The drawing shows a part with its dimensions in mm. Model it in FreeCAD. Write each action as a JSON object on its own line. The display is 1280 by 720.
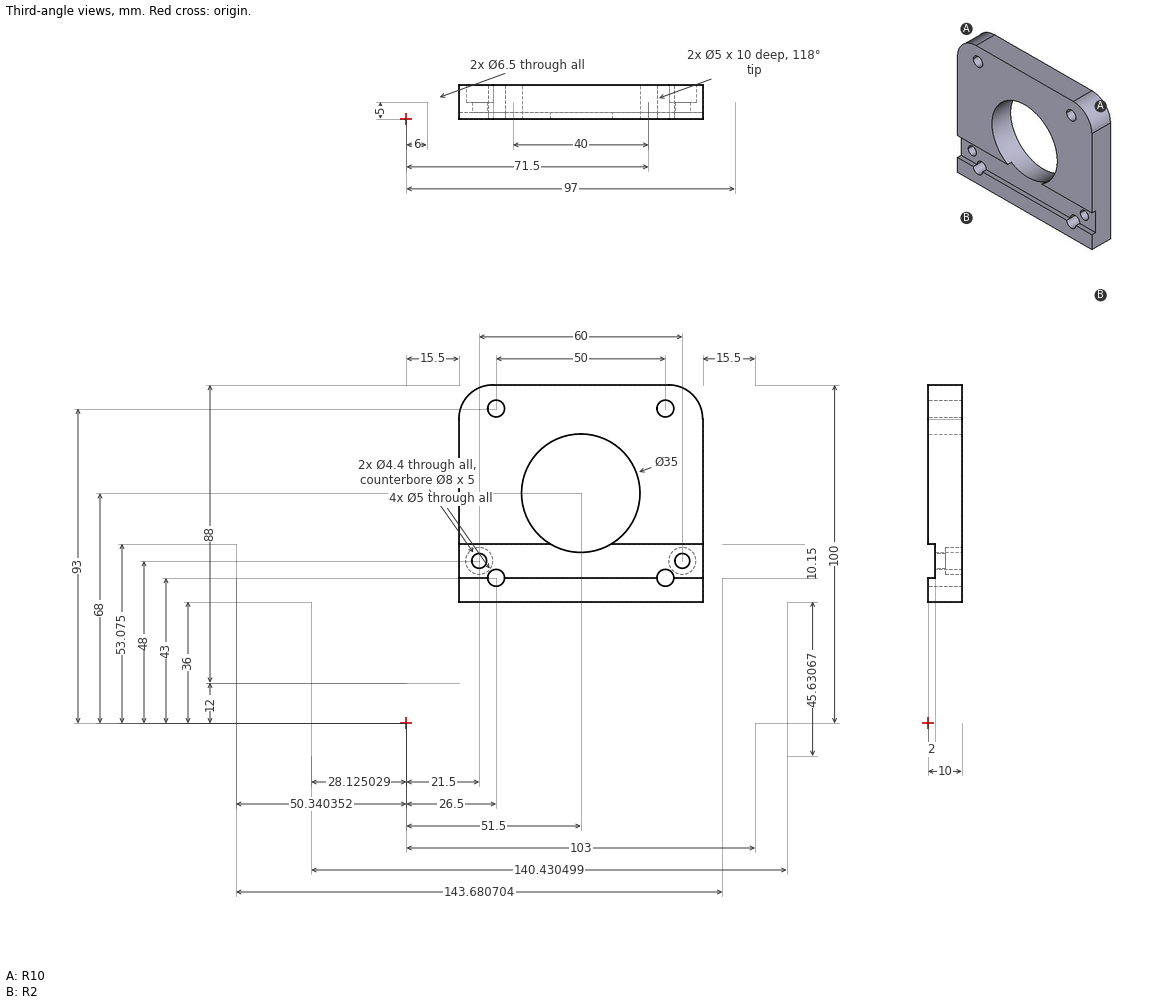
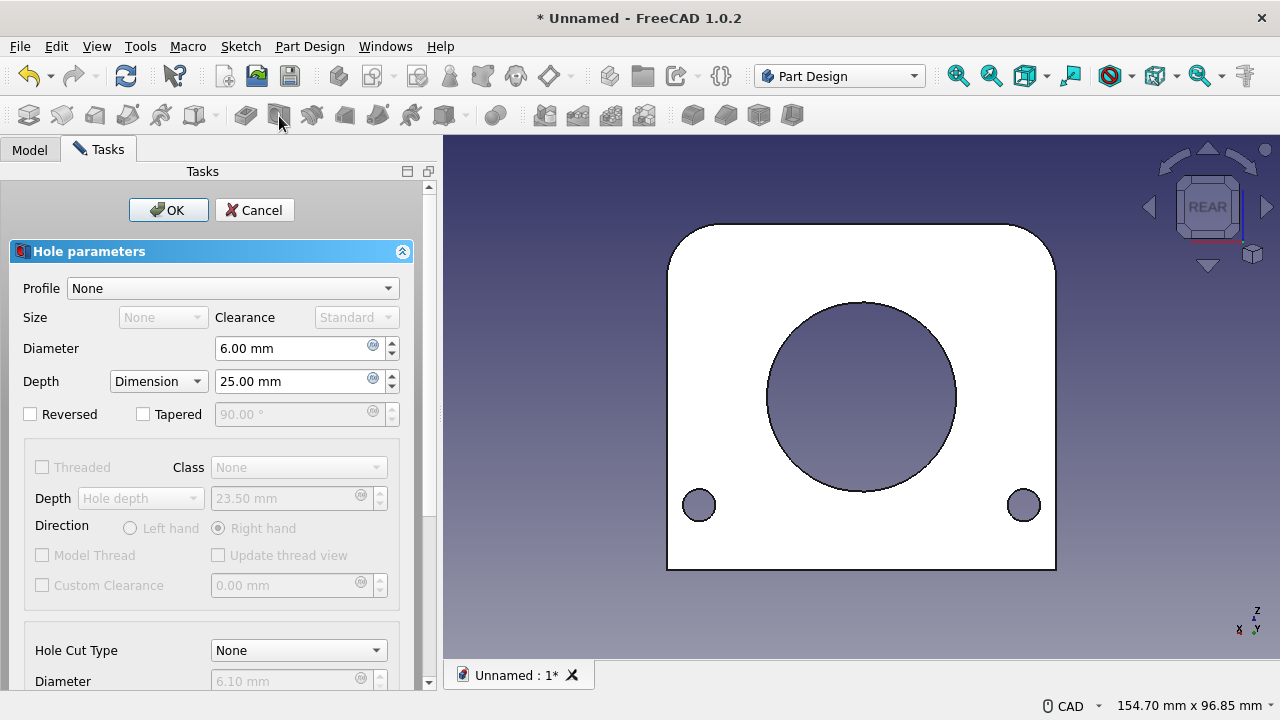
{"action": "triple_click", "coordinate": [300, 348]}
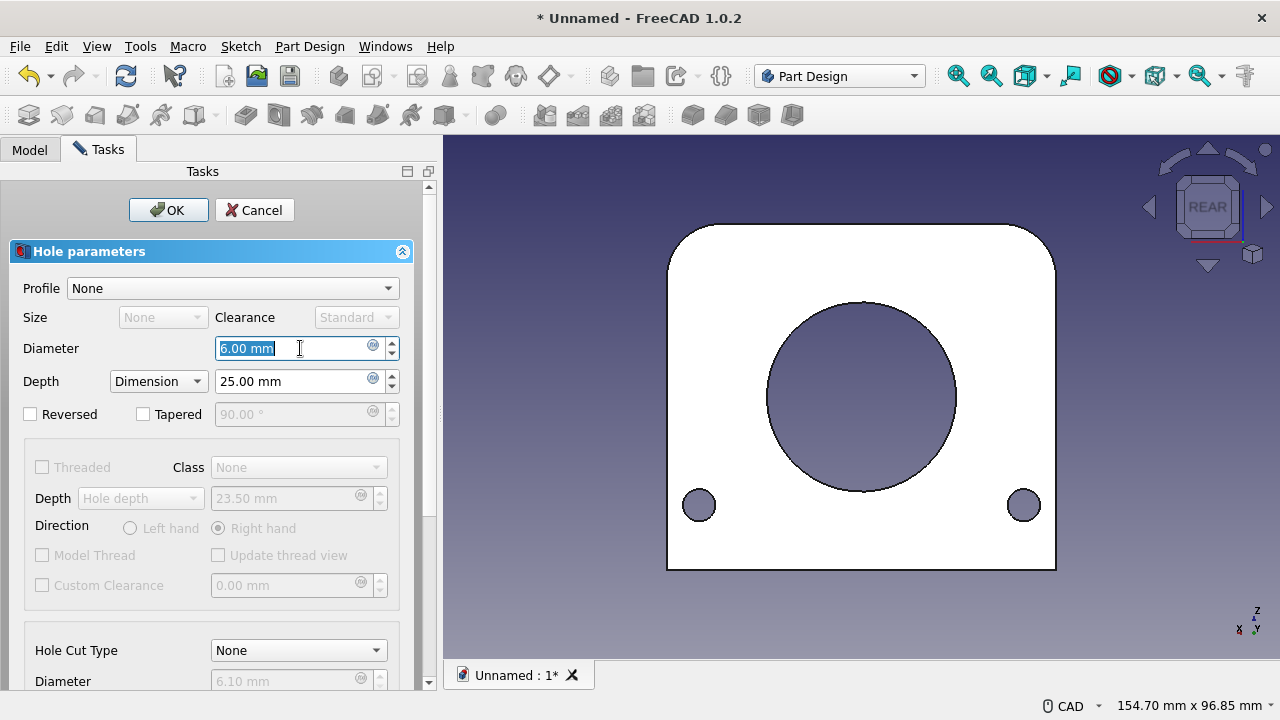
{"action": "type", "text": "4.4"}
{"action": "key", "text": "Tab"}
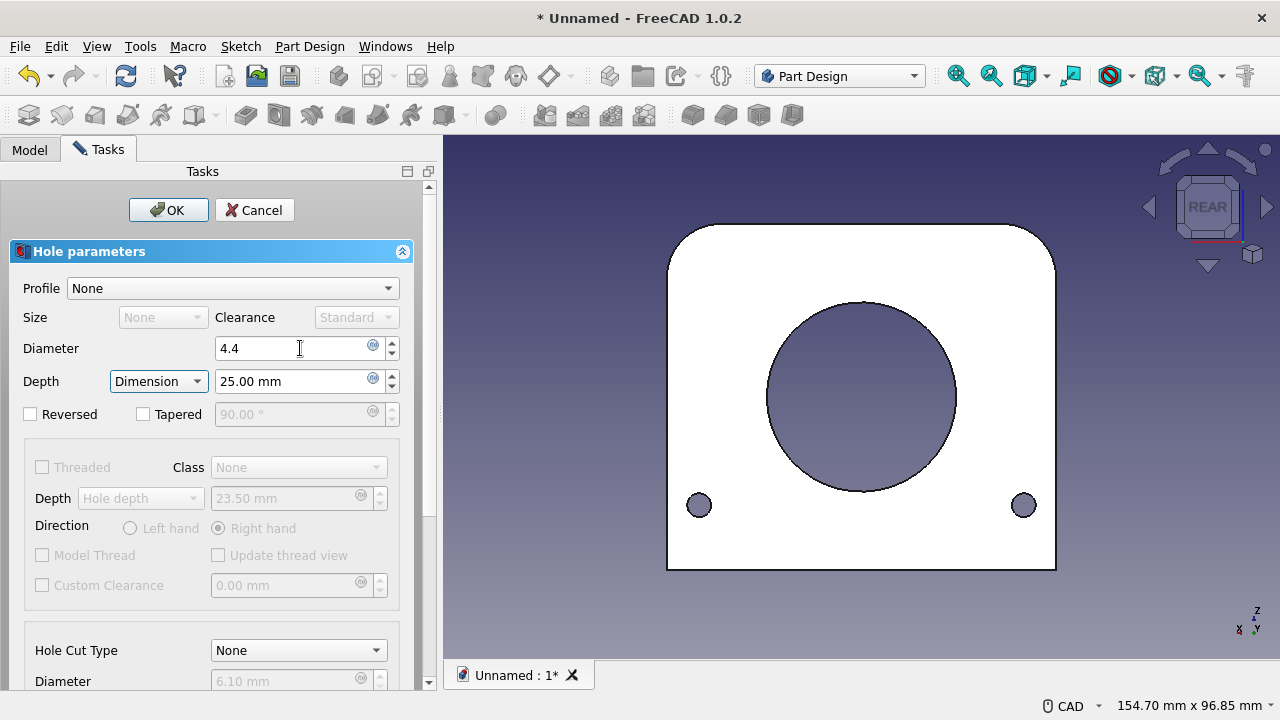
{"action": "left_click", "coordinate": [160, 382]}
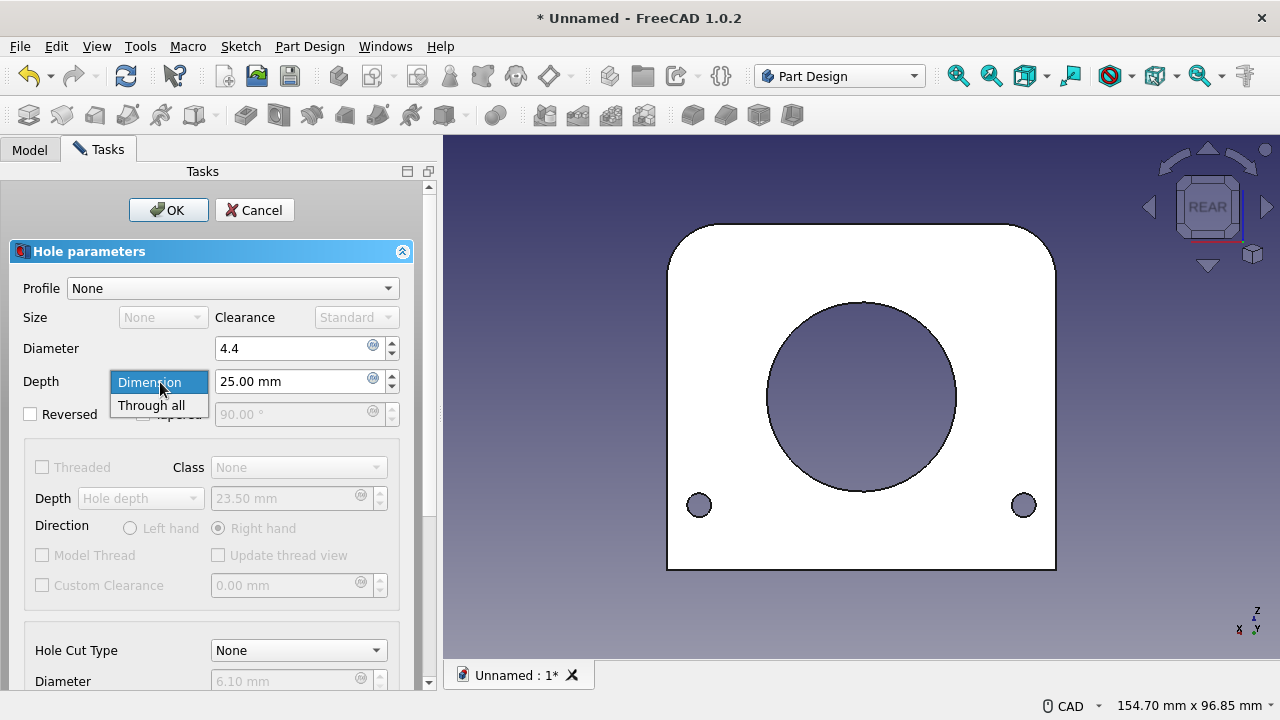
{"action": "left_click", "coordinate": [158, 406]}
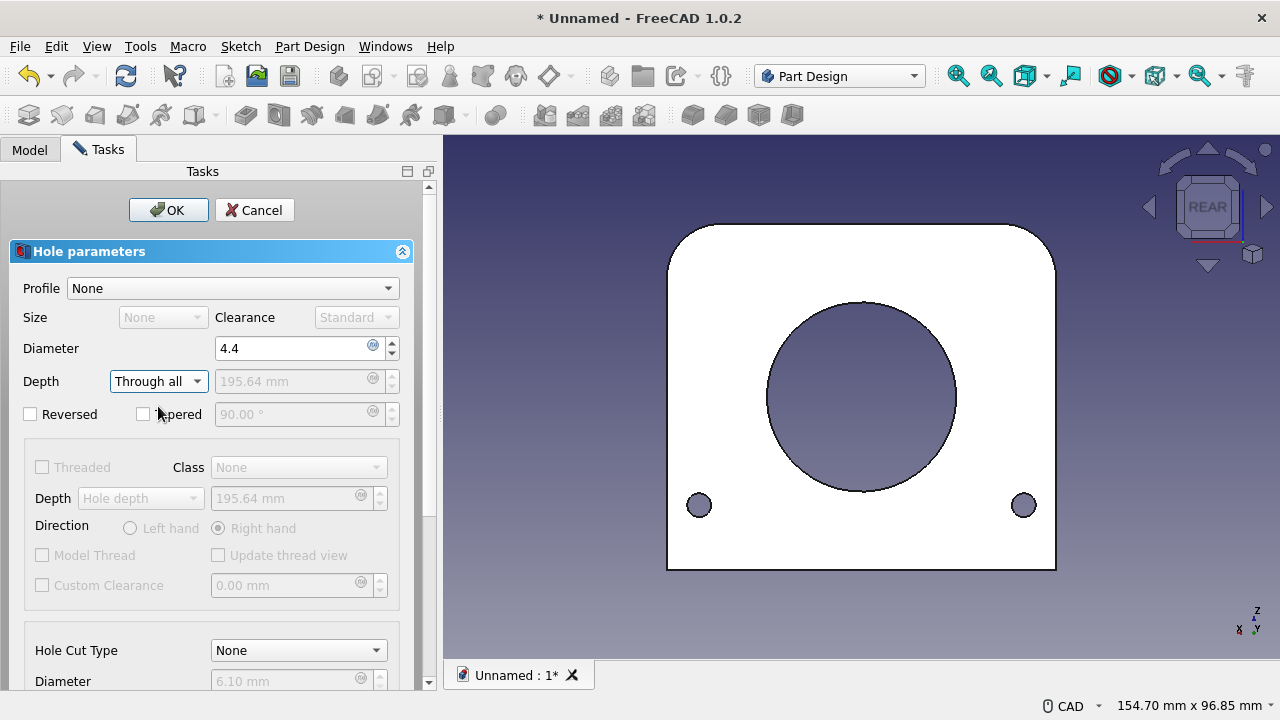
{"action": "left_click", "coordinate": [300, 650]}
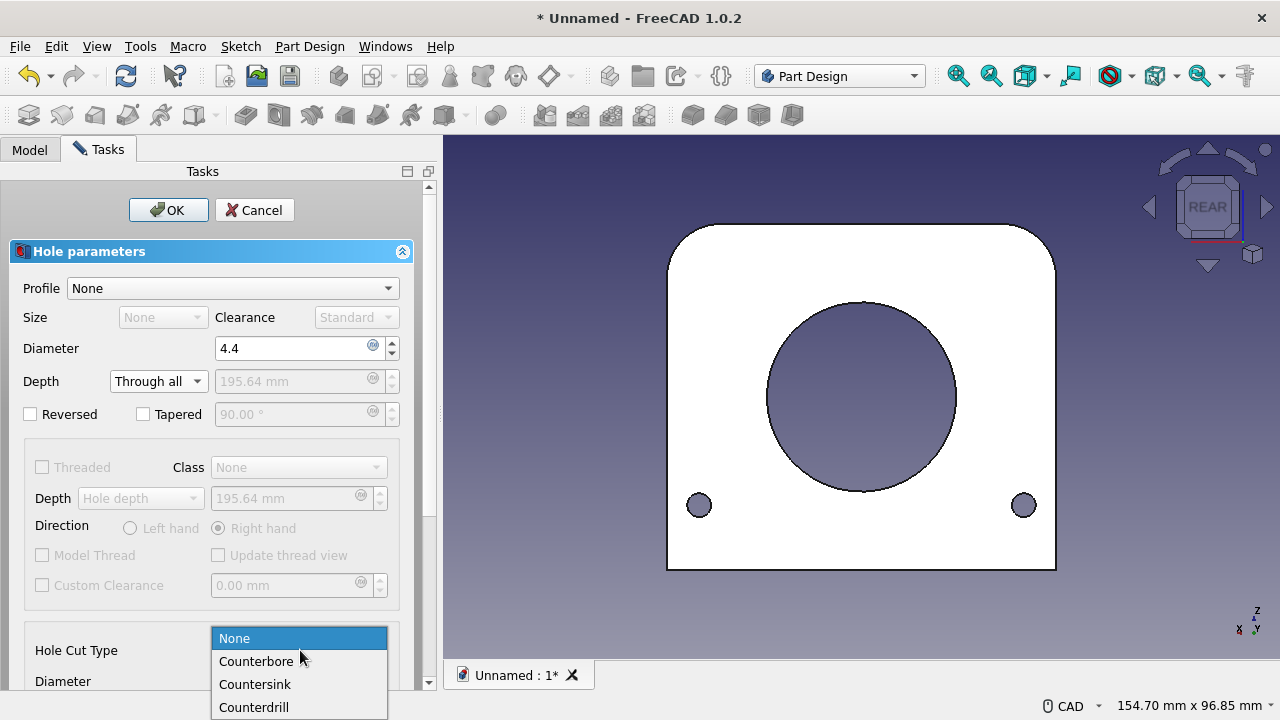
{"action": "left_click", "coordinate": [298, 662]}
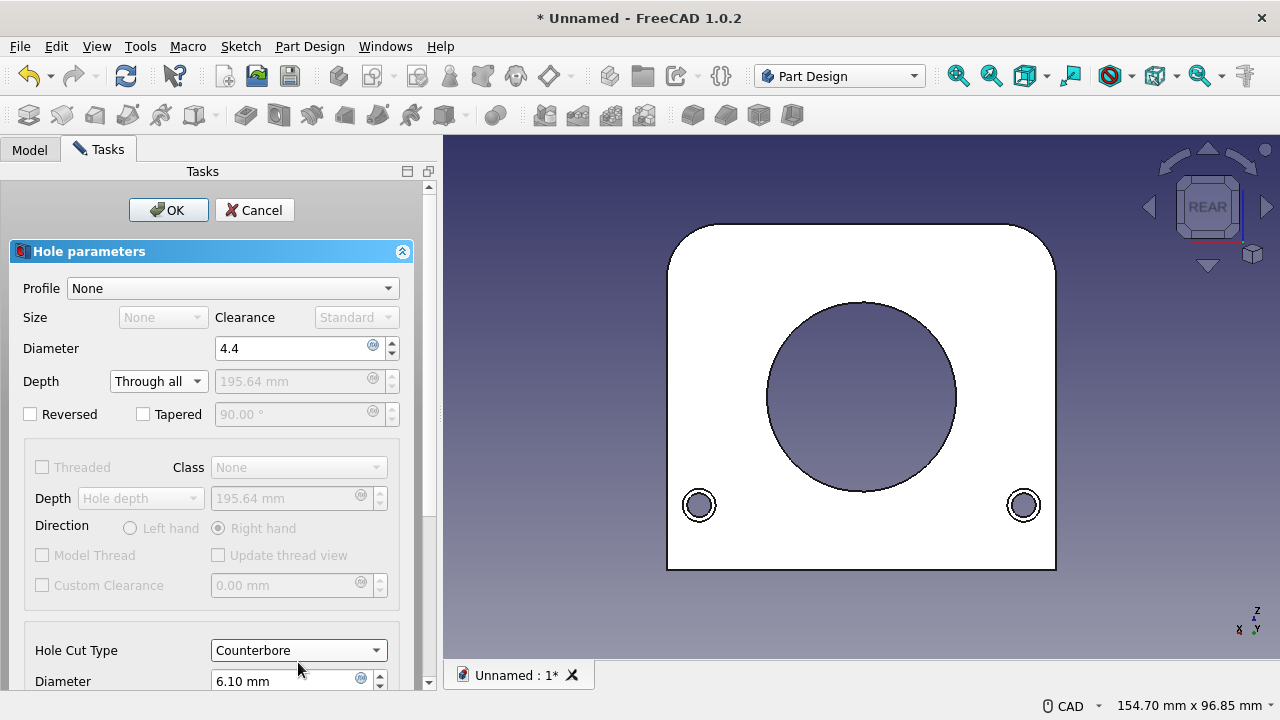
{"action": "scroll", "coordinate": [429, 436], "scroll_direction": "down", "scroll_amount": 2}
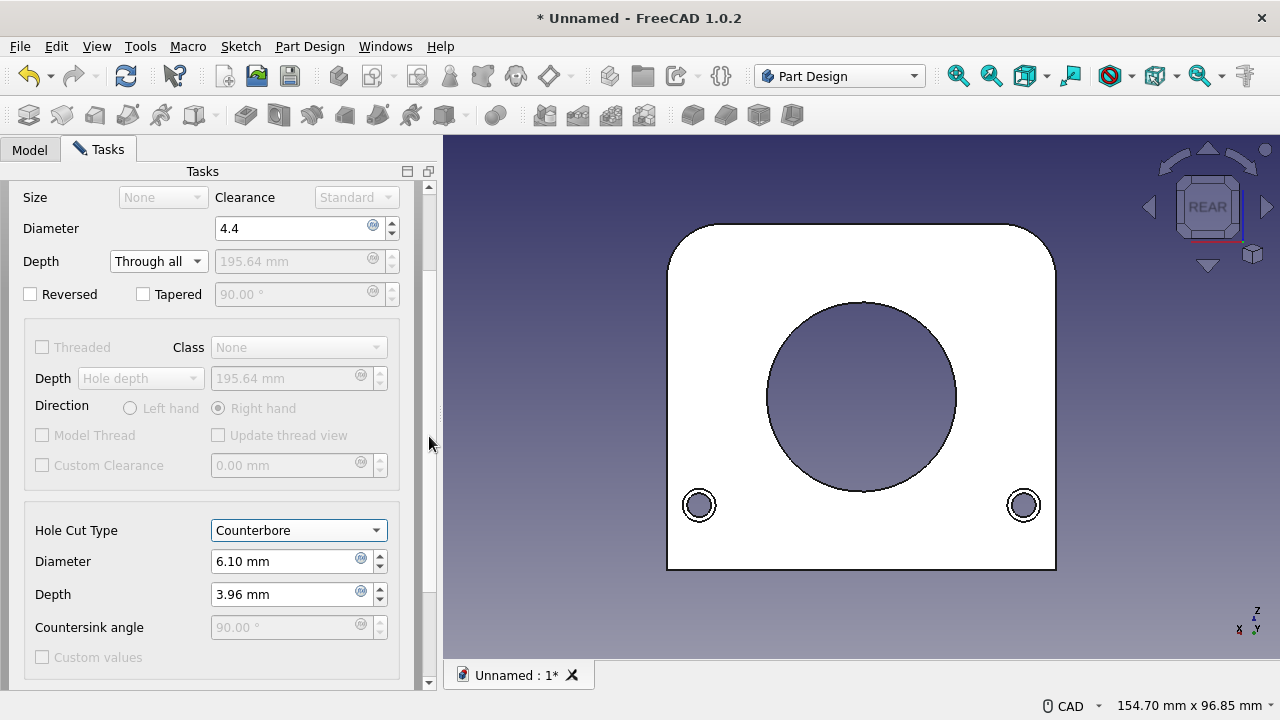
{"action": "triple_click", "coordinate": [292, 562]}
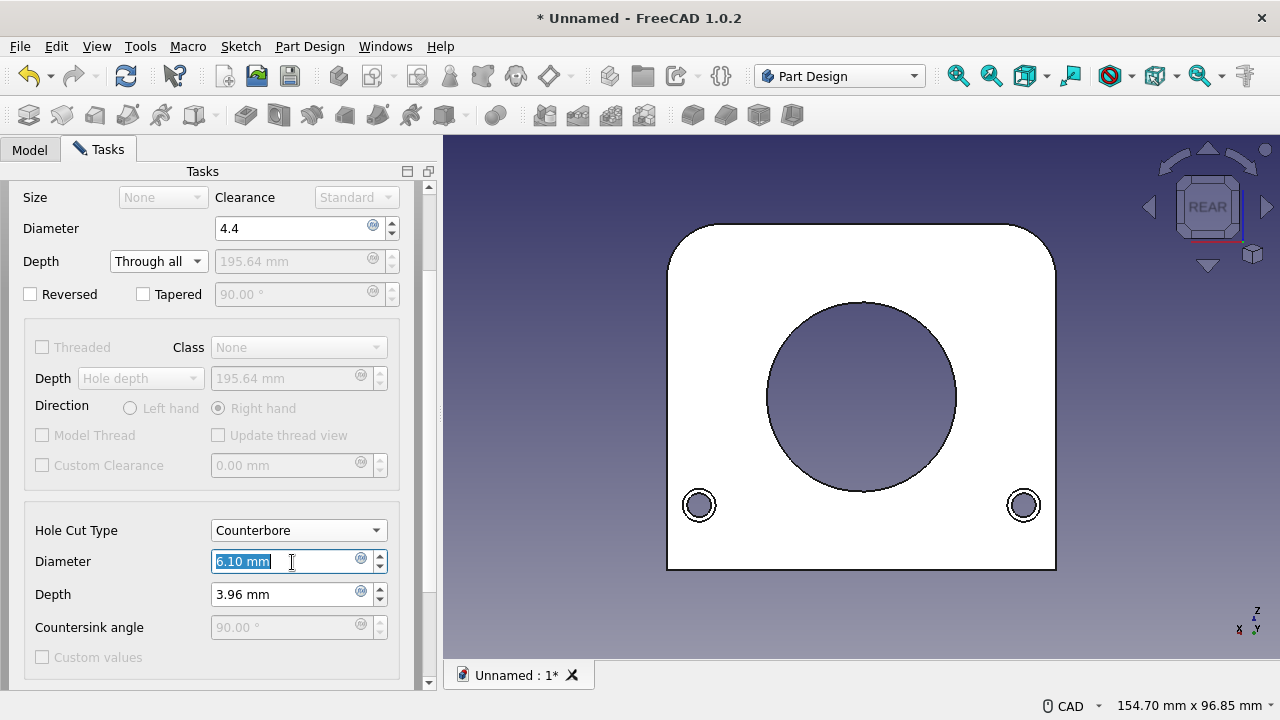
{"action": "type", "text": "8"}
{"action": "key", "text": "Tab"}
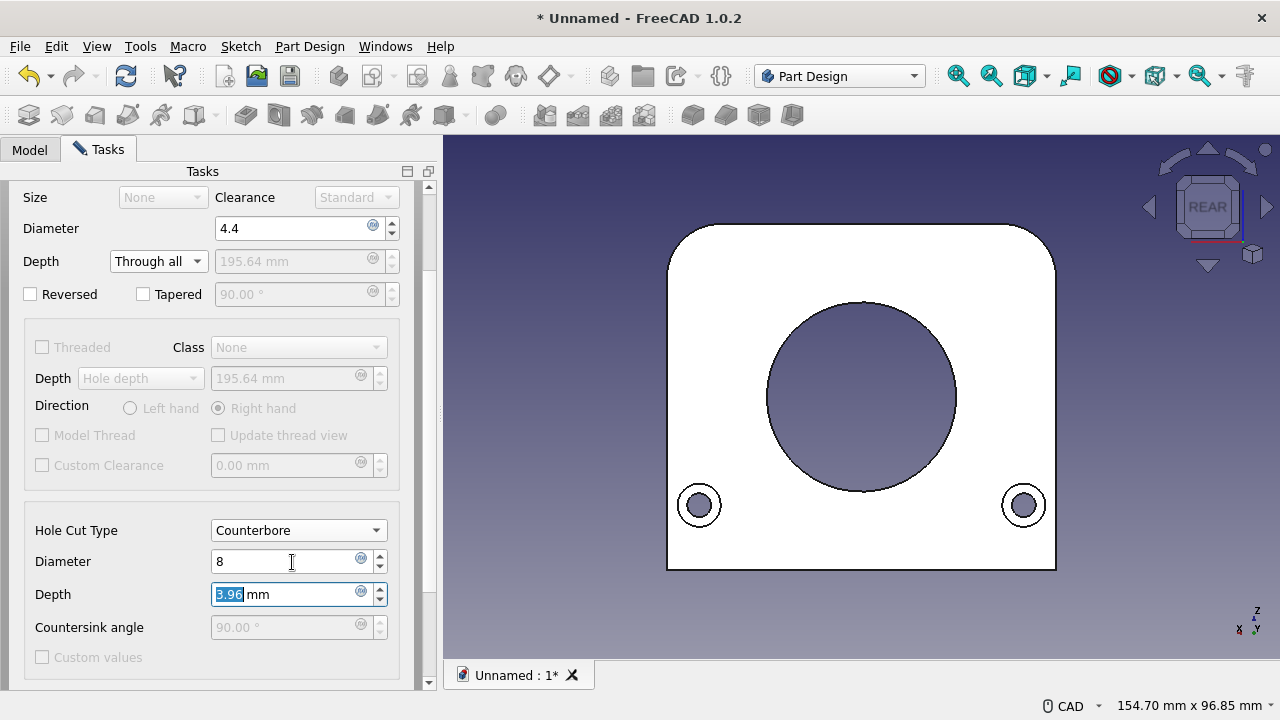
{"action": "type", "text": "5"}
{"action": "key", "text": "Tab"}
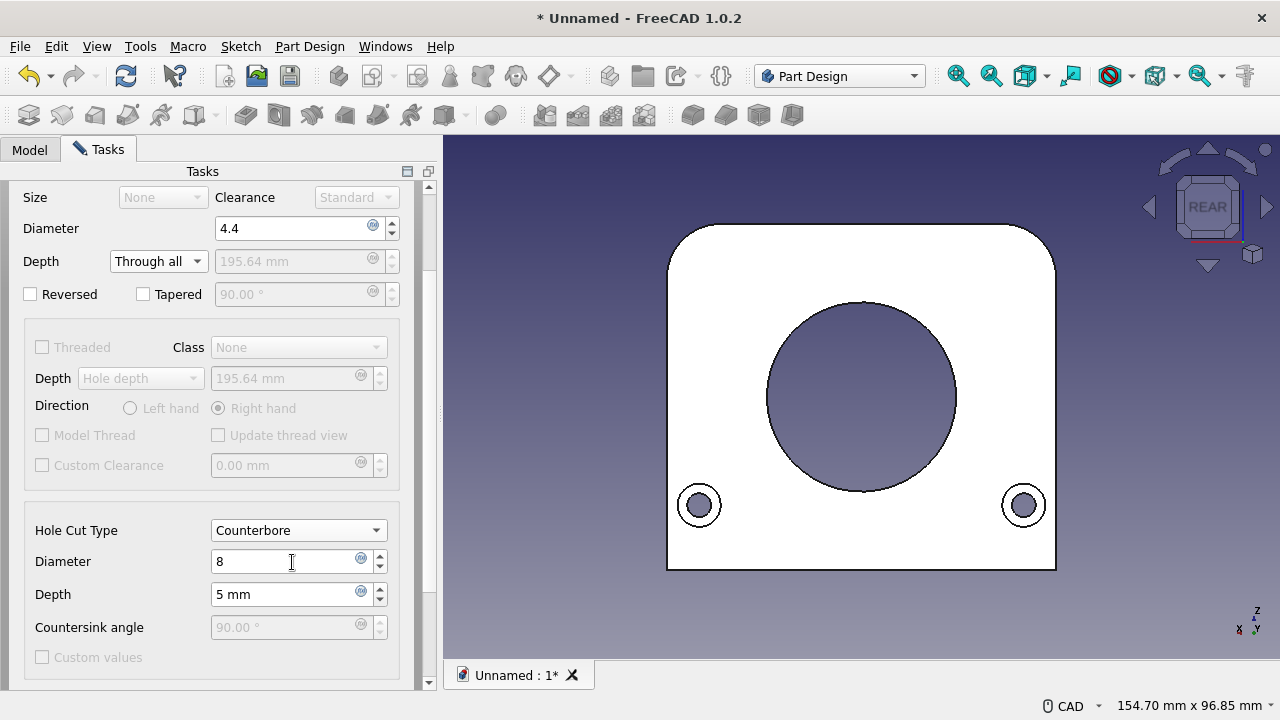
{"action": "scroll", "coordinate": [429, 436], "scroll_direction": "up", "scroll_amount": 3}